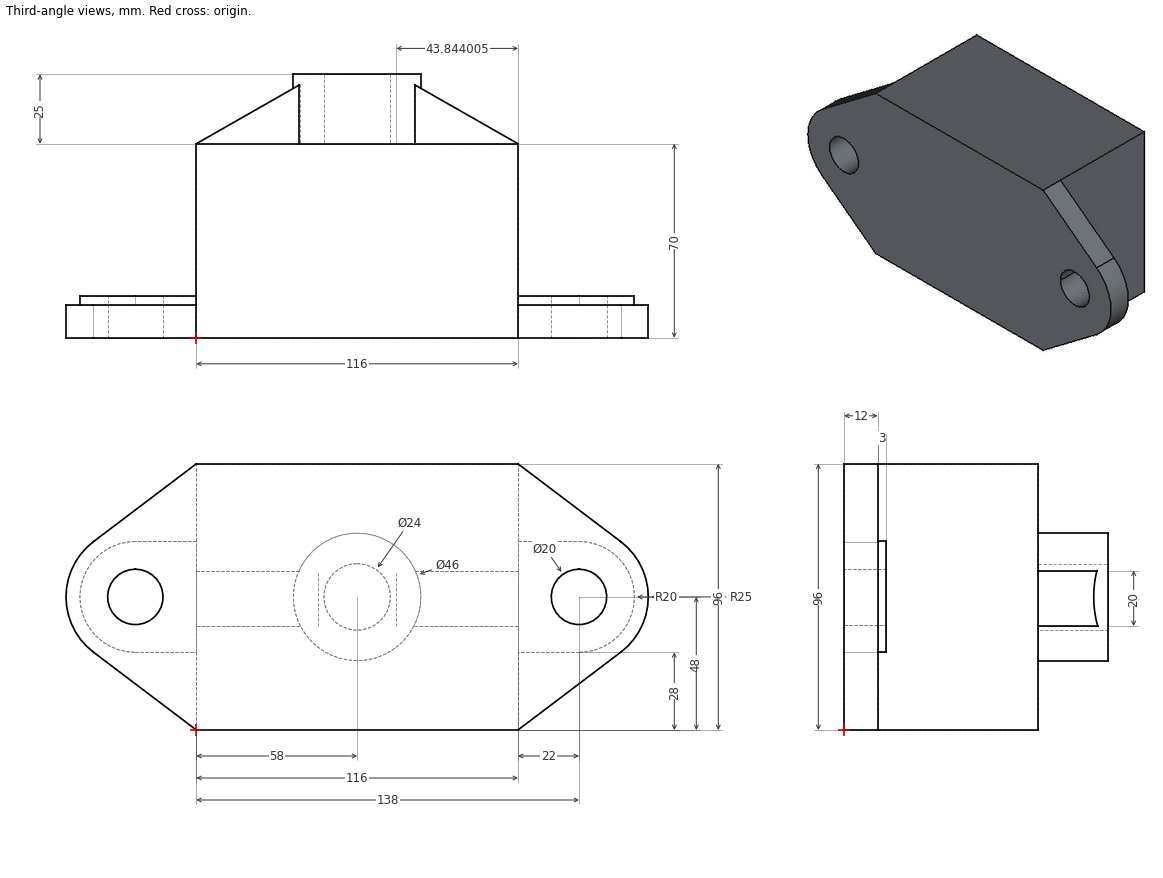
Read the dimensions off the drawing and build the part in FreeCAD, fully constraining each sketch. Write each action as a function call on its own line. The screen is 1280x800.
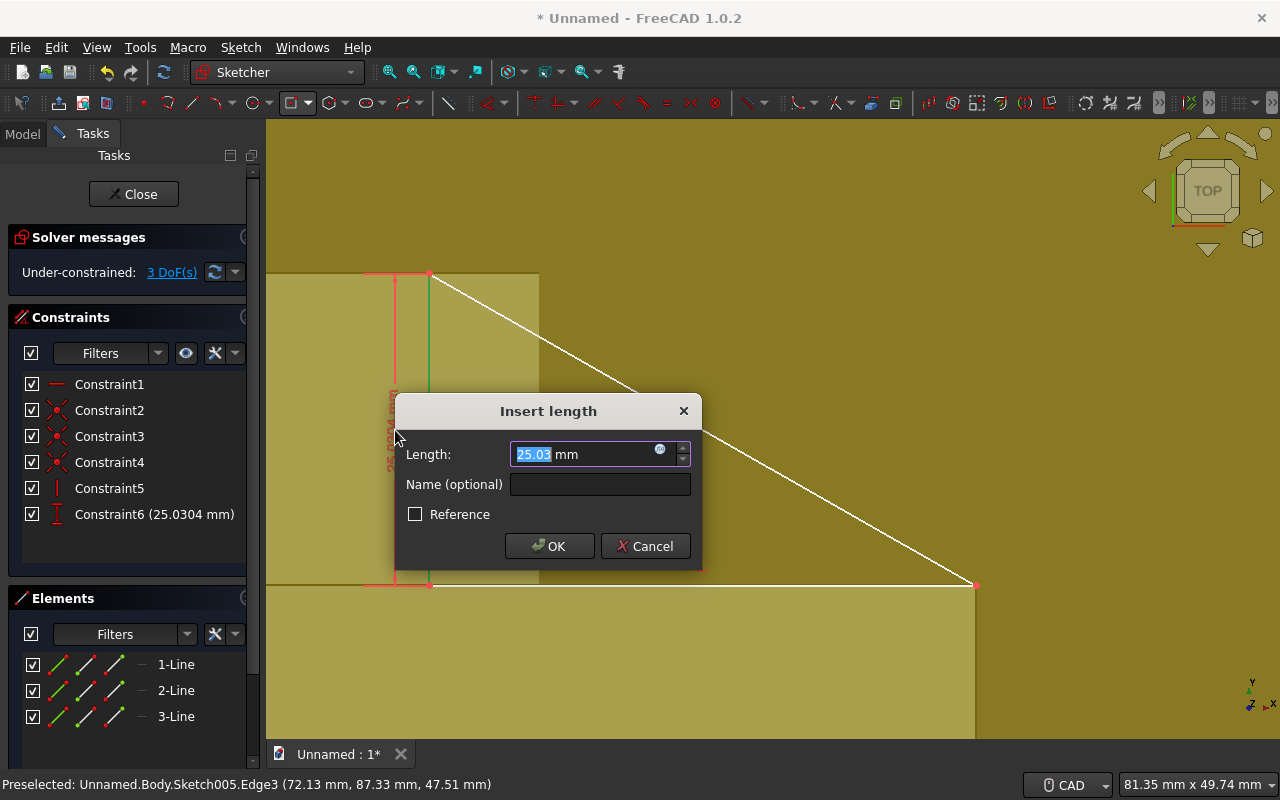
text(25)
key(Return)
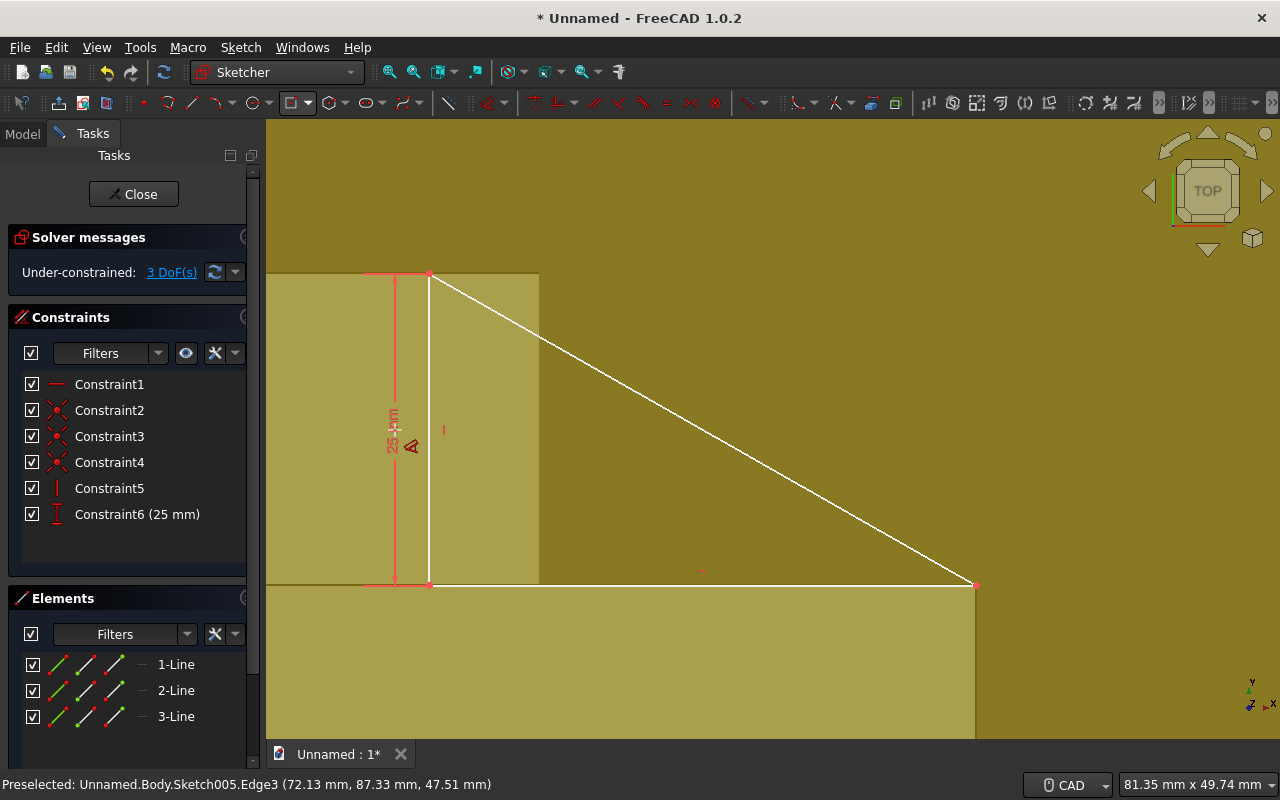
click(429, 586)
click(463, 648)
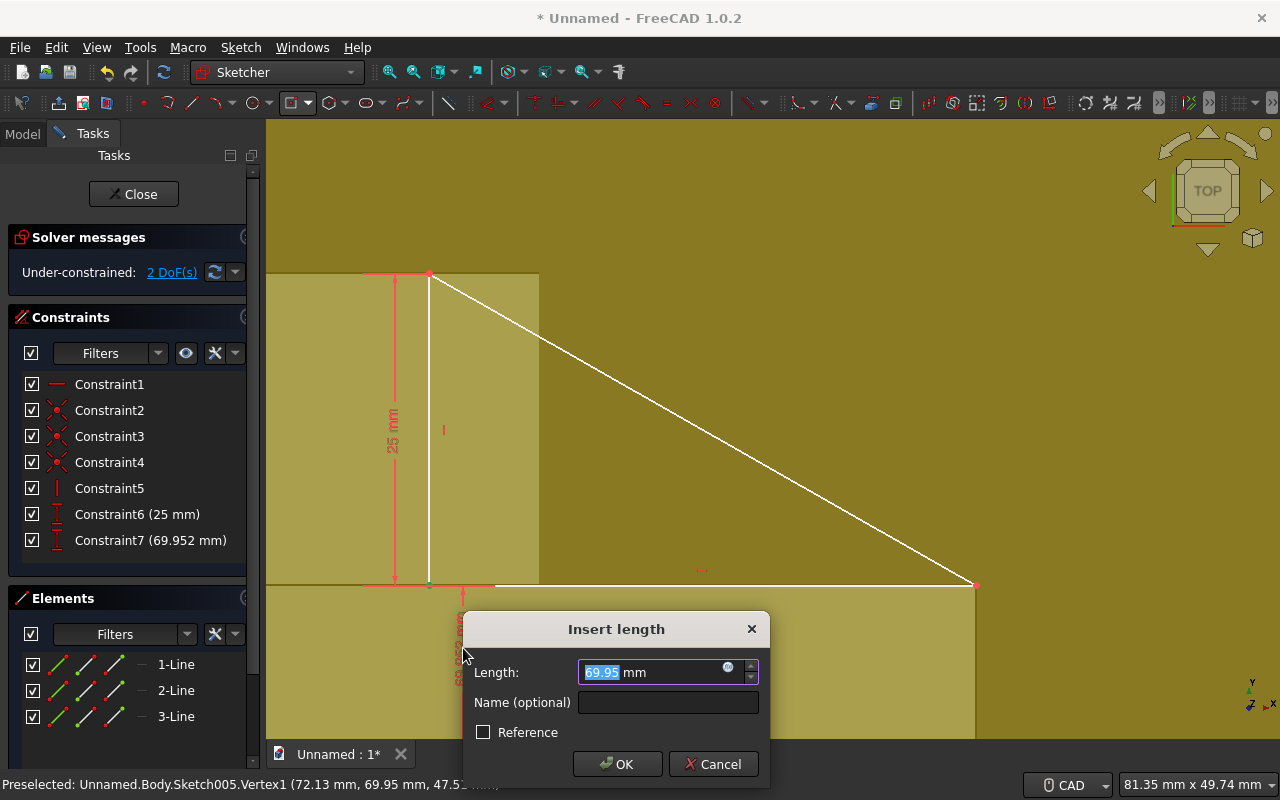
text(70)
key(Return)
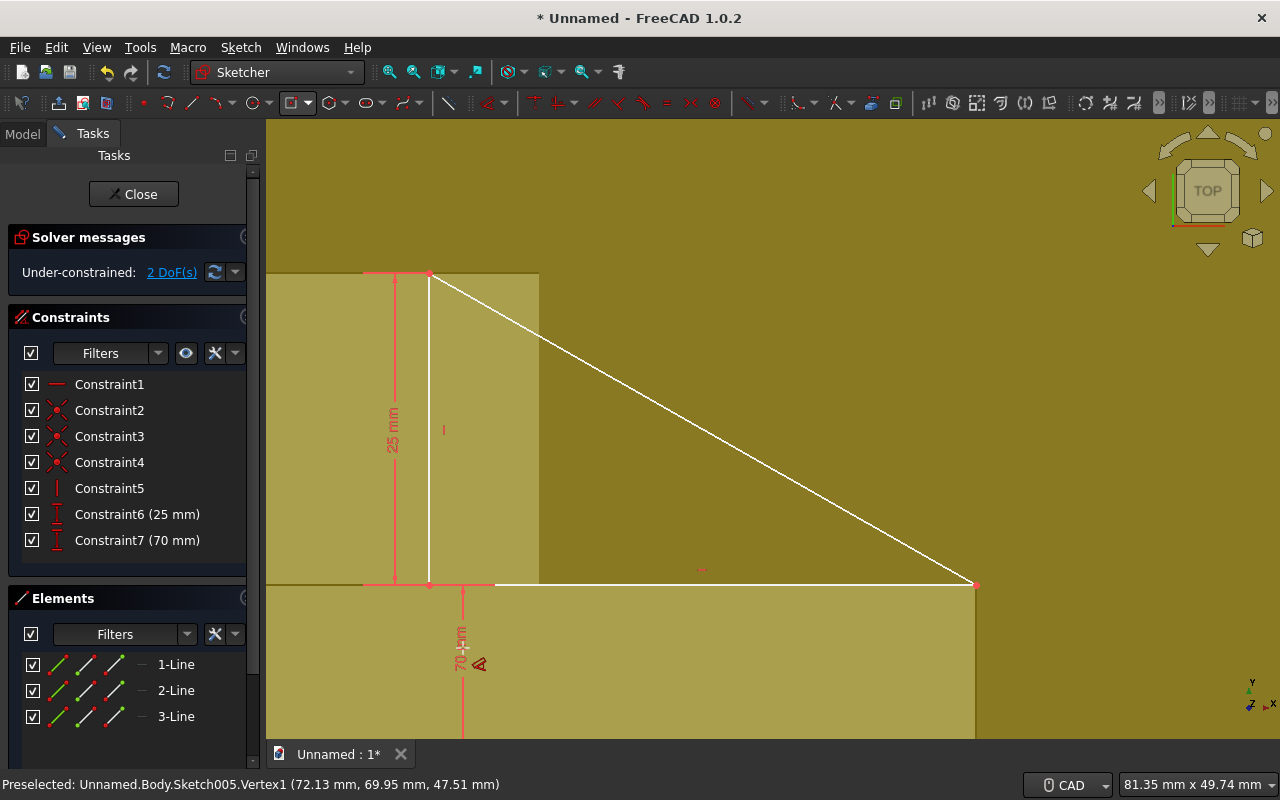
click(976, 585)
click(635, 551)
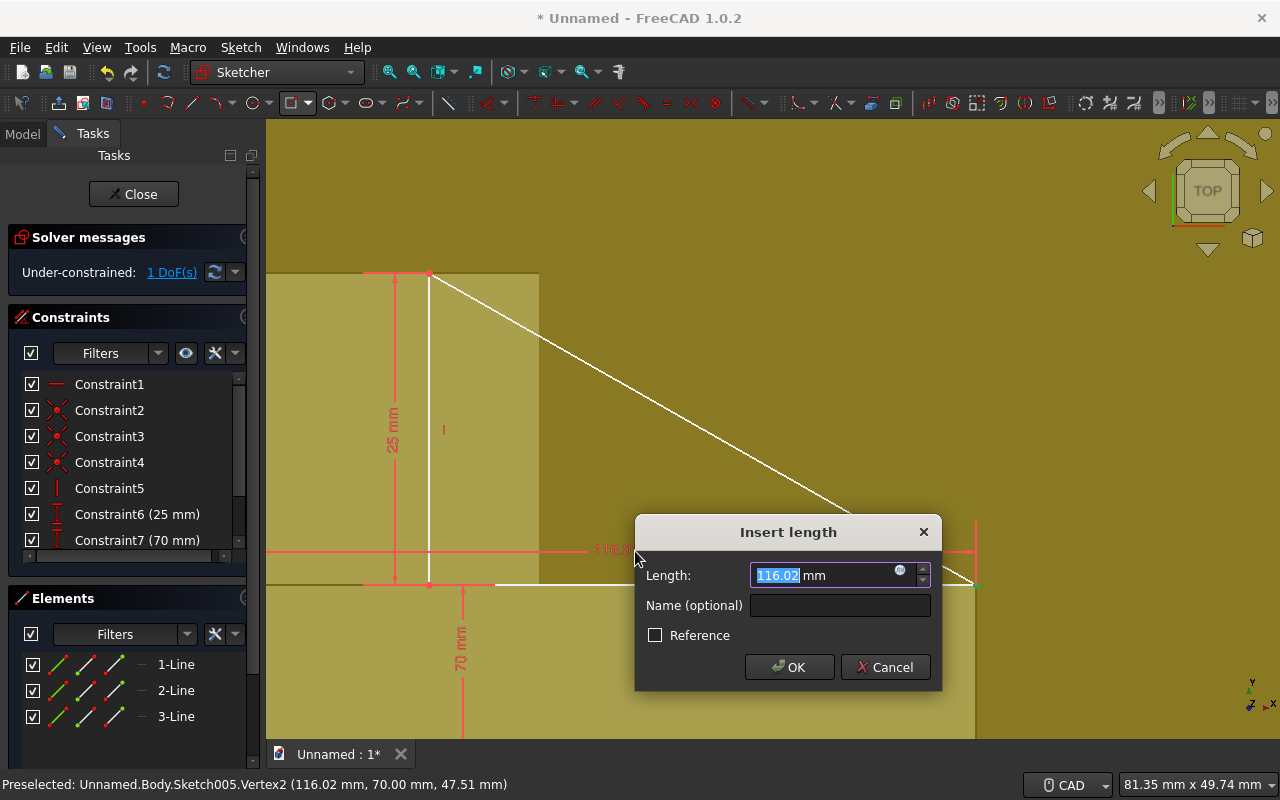
text(116)
key(Return)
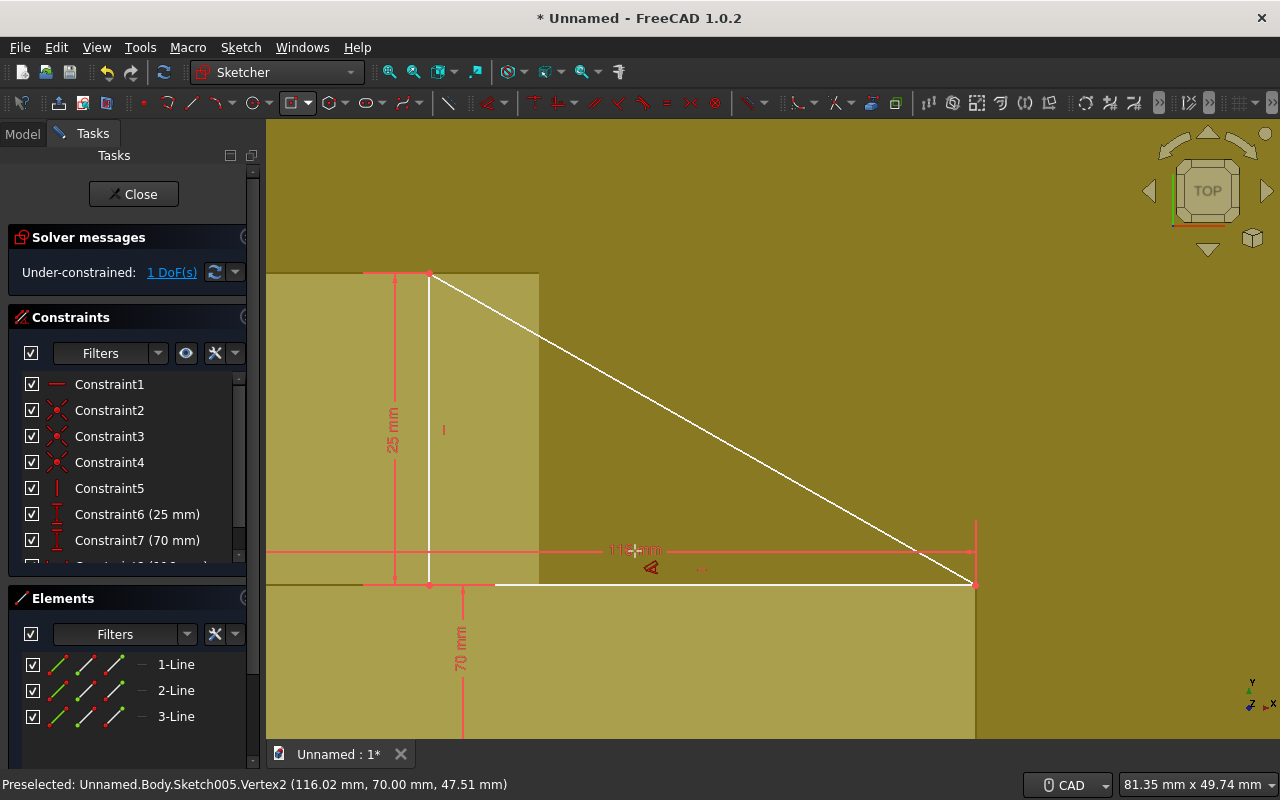
click(593, 585)
click(702, 619)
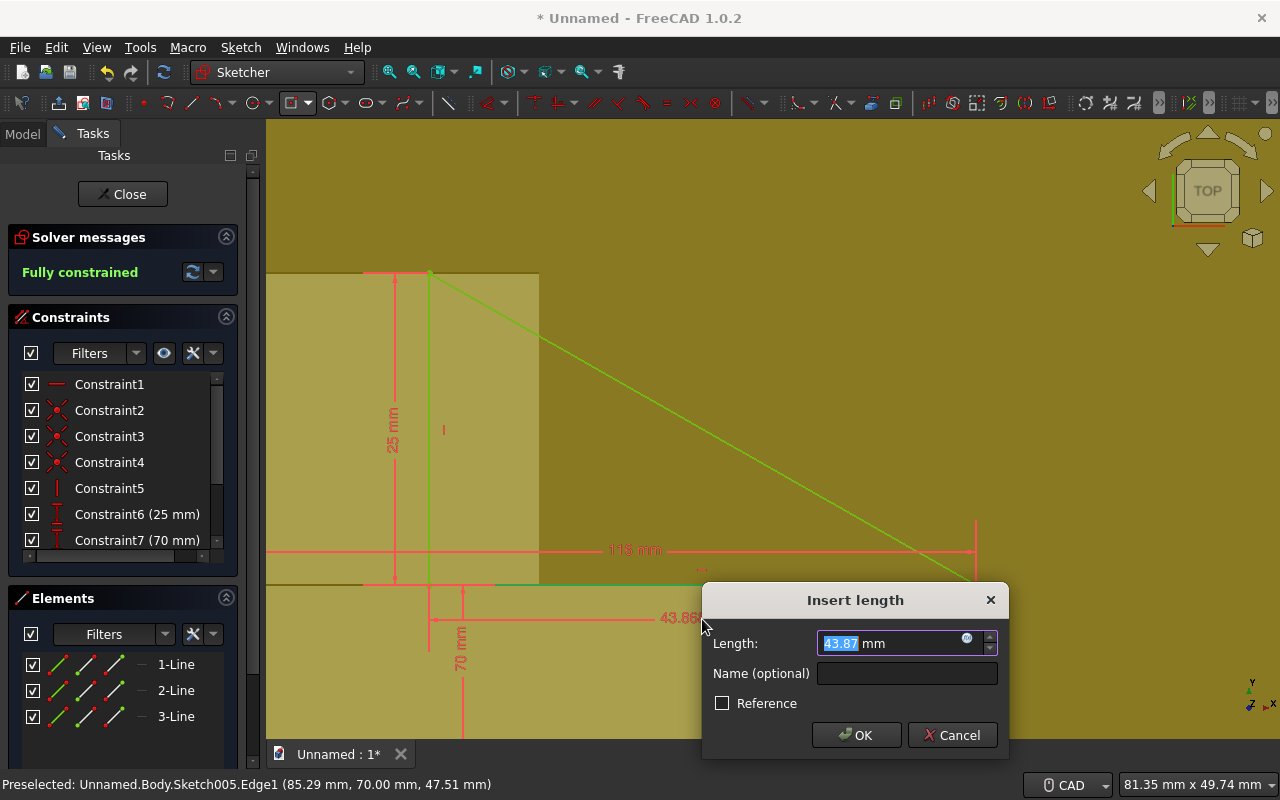
text(43.844005)
key(Return)
key(Escape)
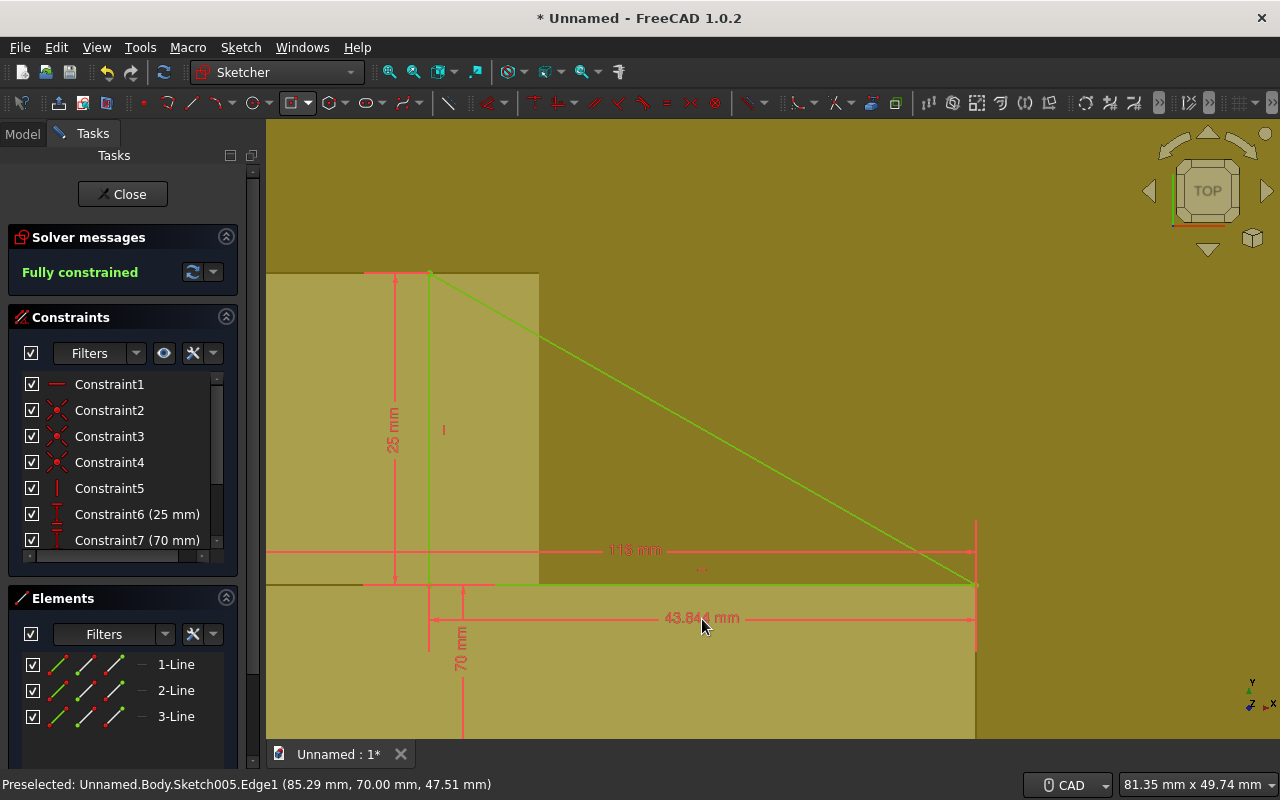
click(123, 194)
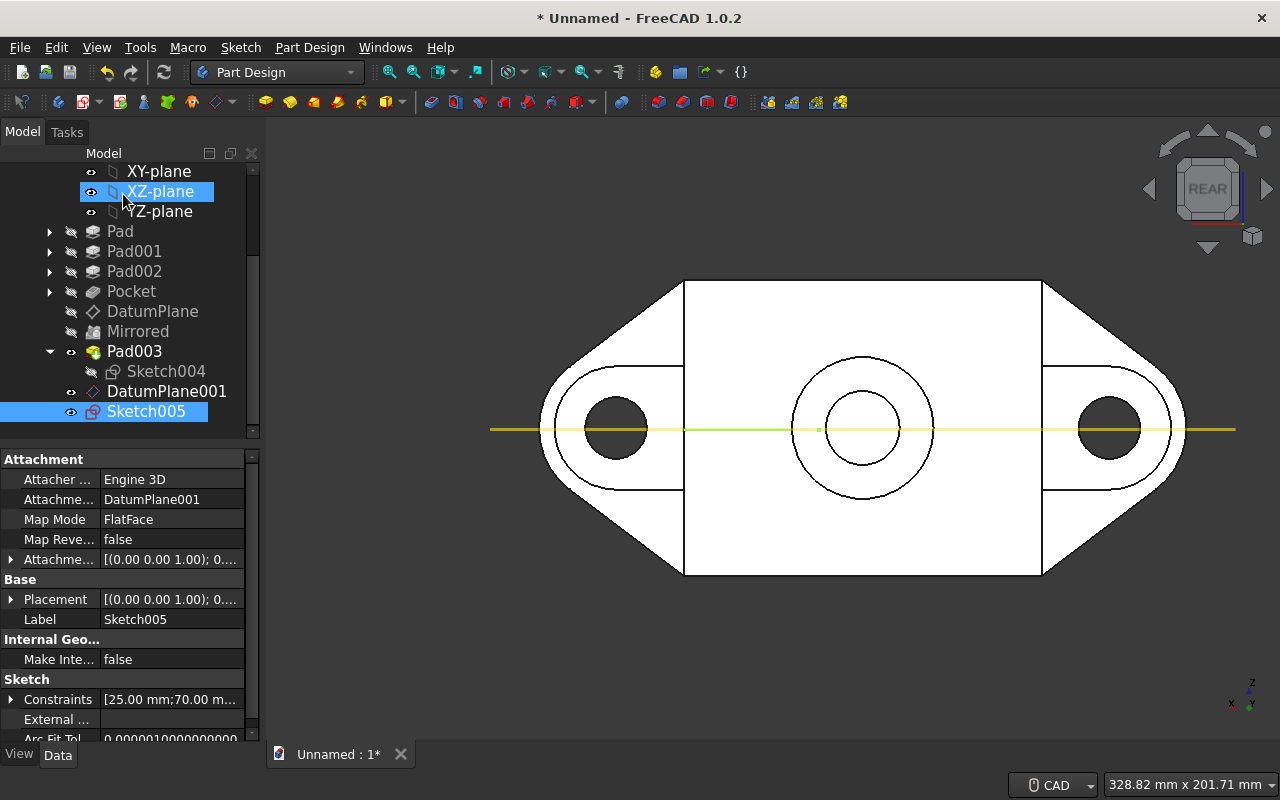
click(266, 102)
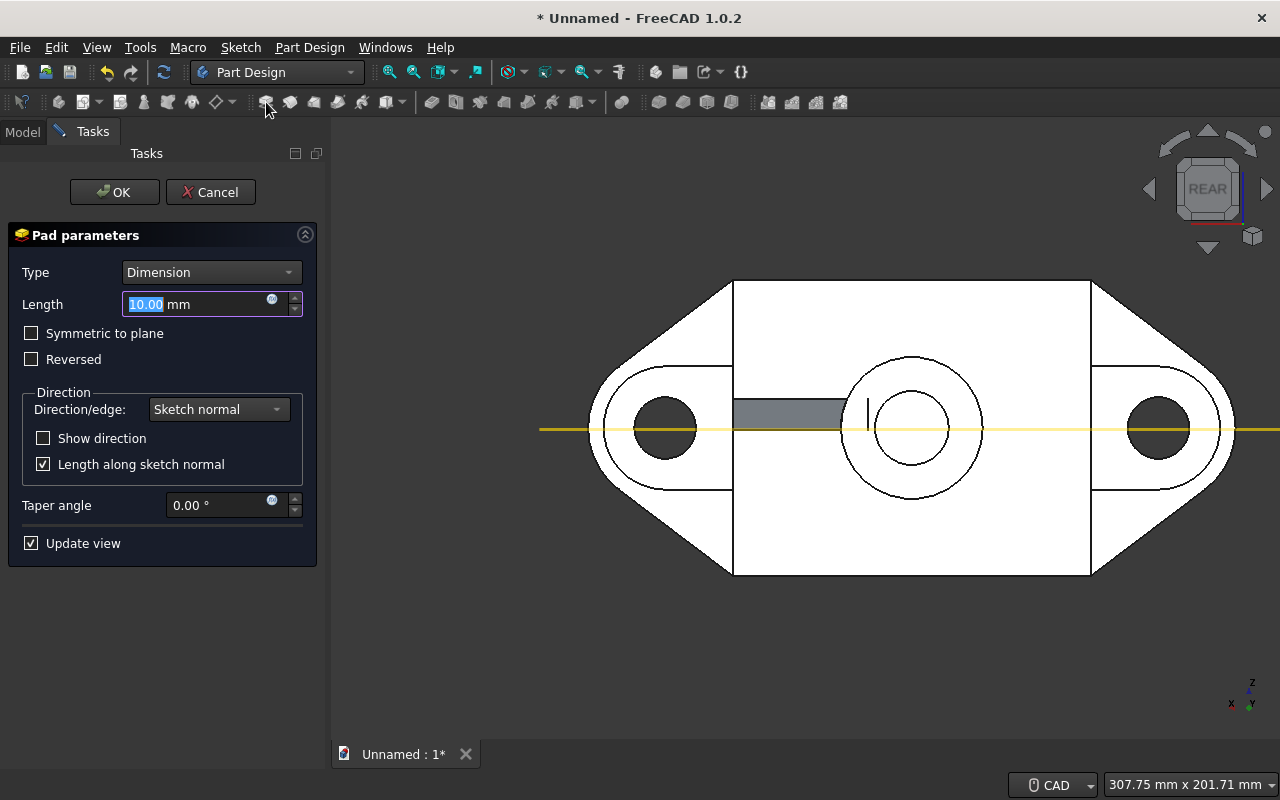
text(20)
key(Tab)